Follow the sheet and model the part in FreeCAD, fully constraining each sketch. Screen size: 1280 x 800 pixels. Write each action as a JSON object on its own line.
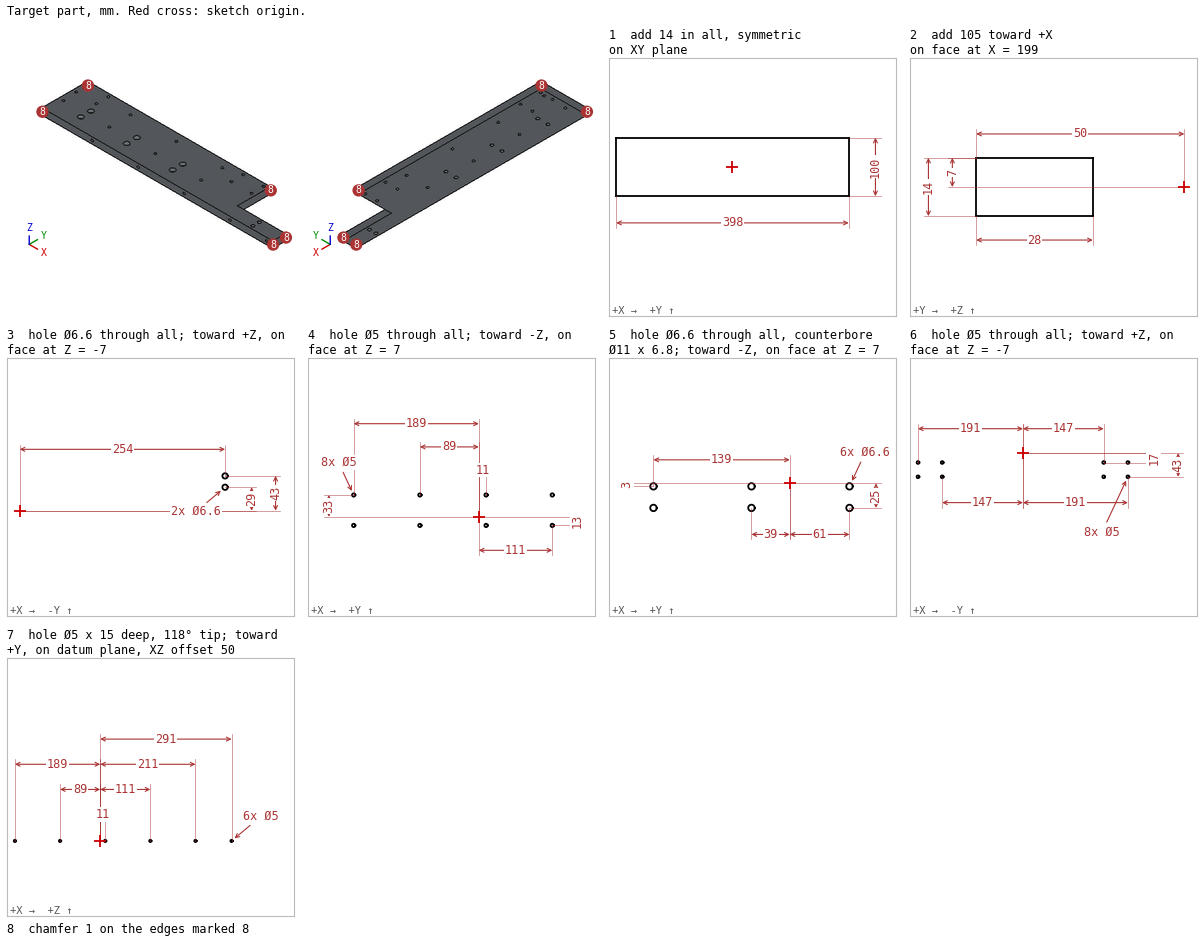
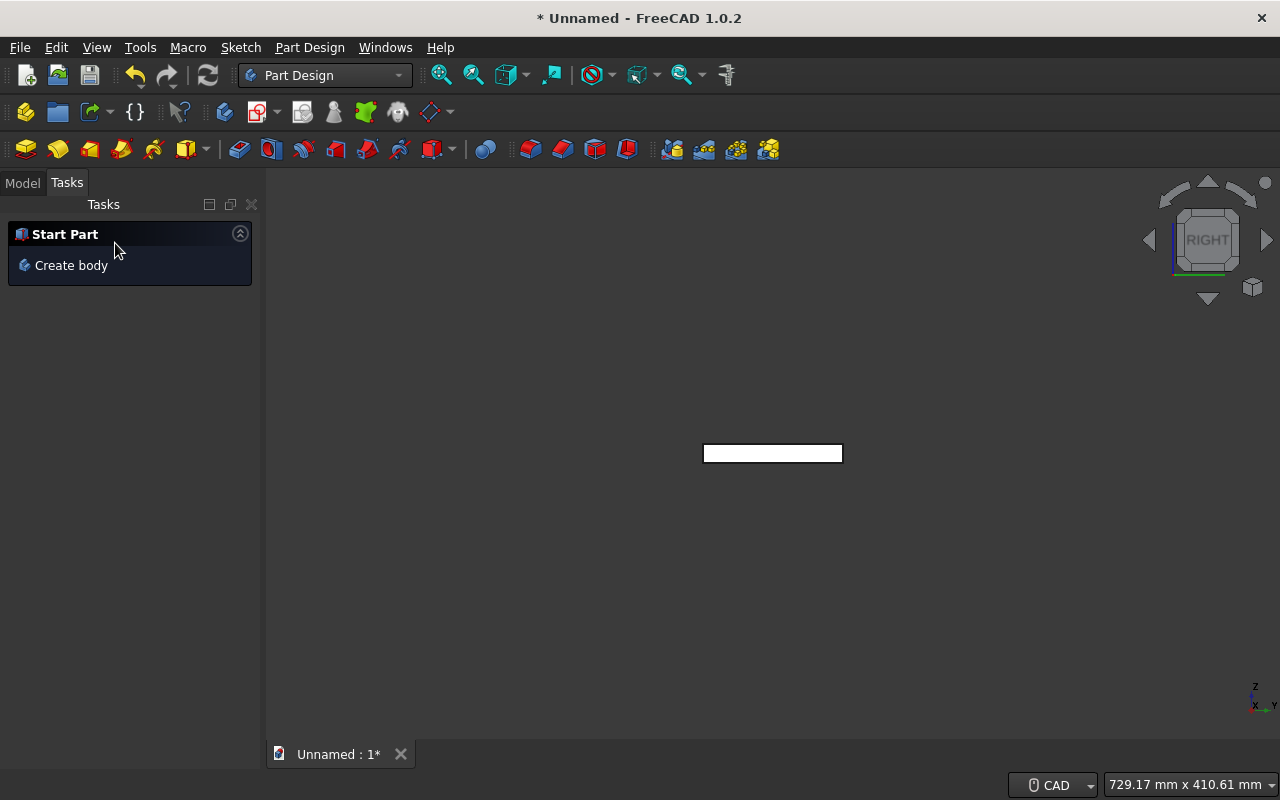
{"action": "key", "text": "v f"}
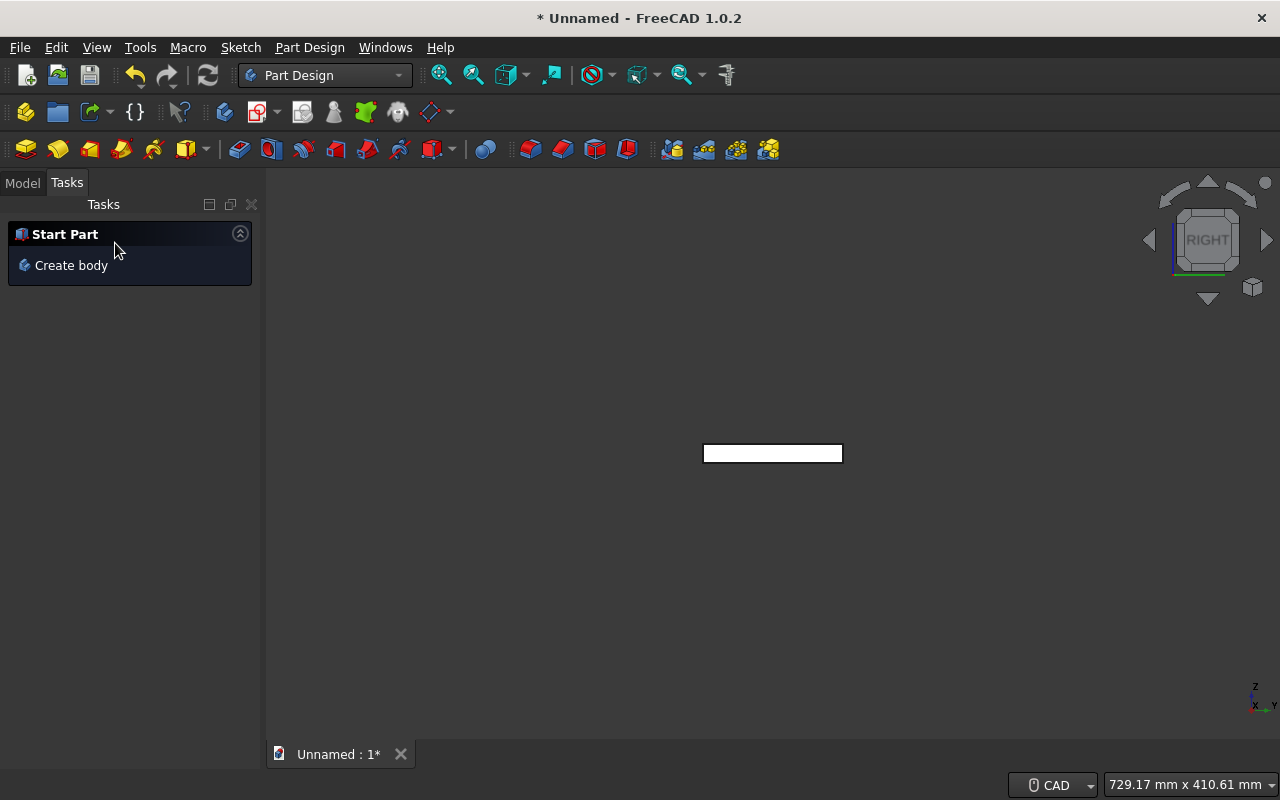
{"action": "left_click", "coordinate": [833, 452]}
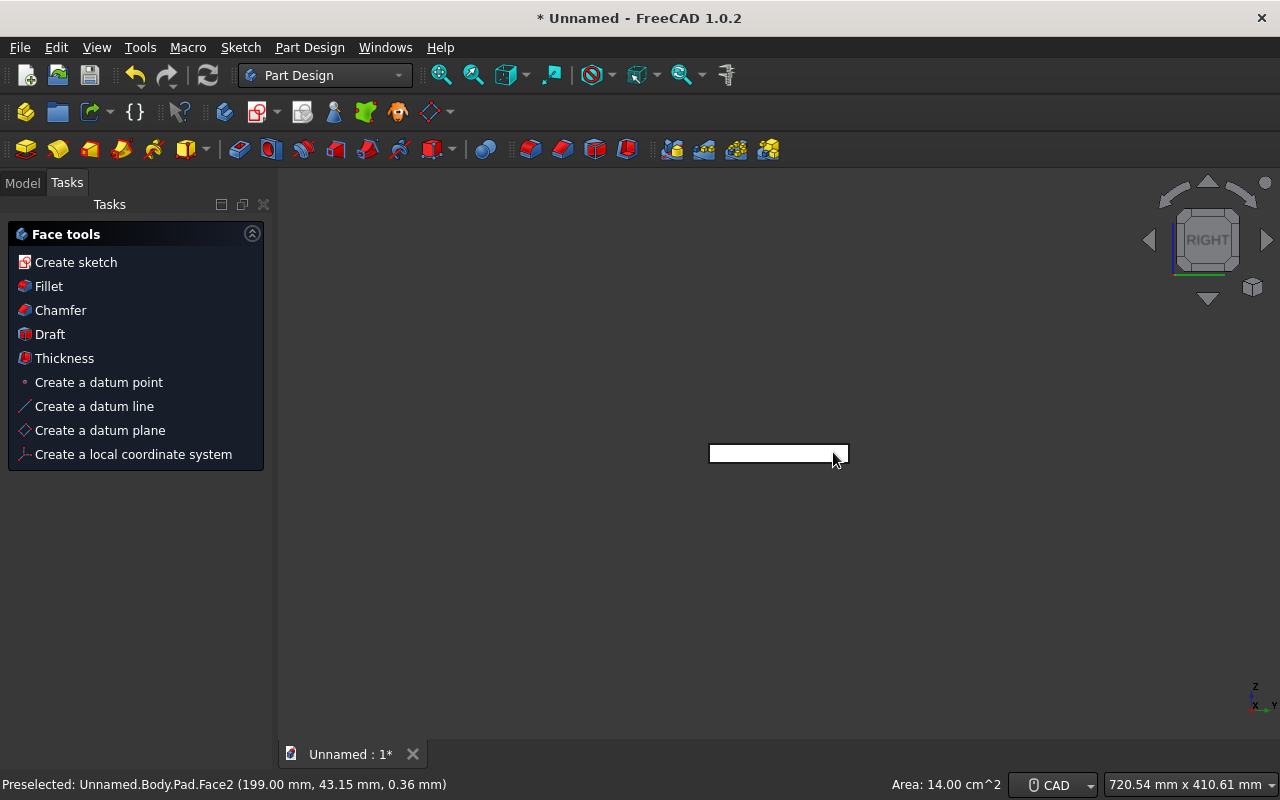
{"action": "left_click", "coordinate": [258, 112]}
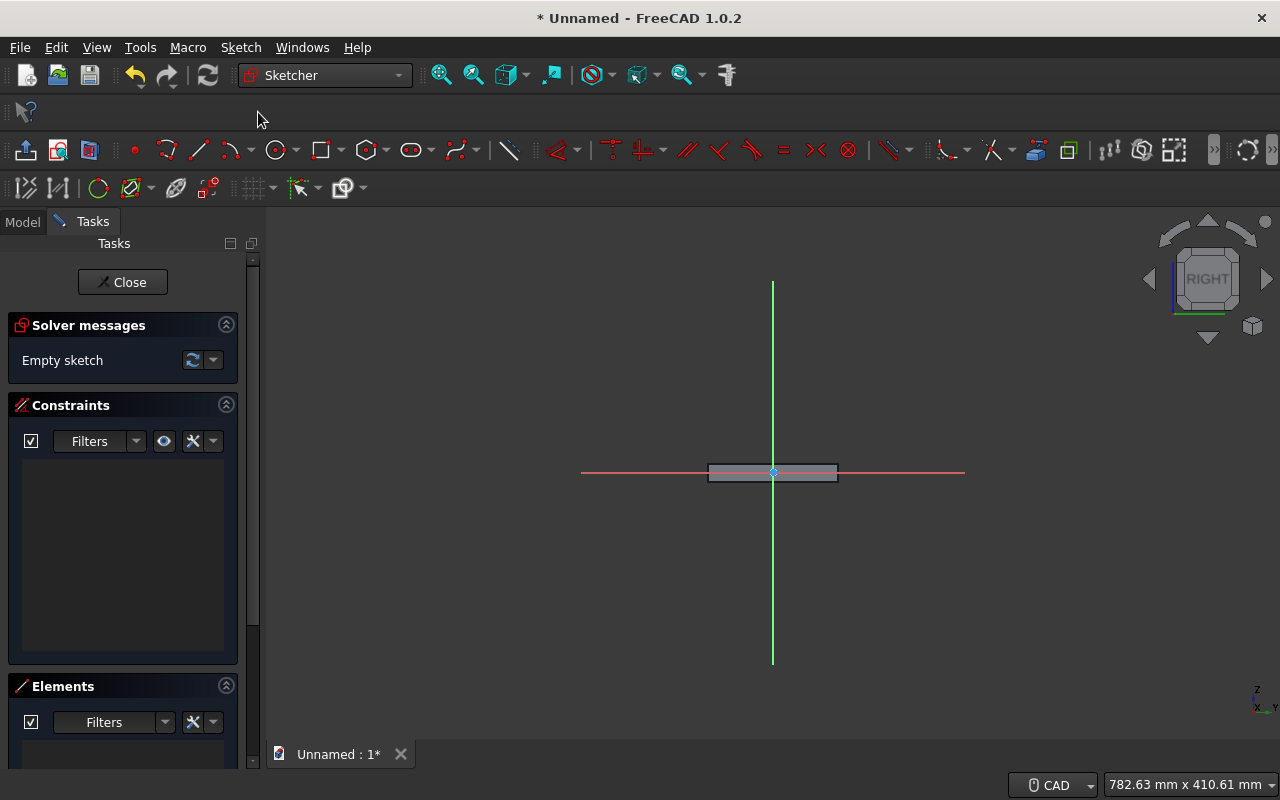
{"action": "scroll", "coordinate": [745, 473], "scroll_direction": "up", "scroll_amount": 11}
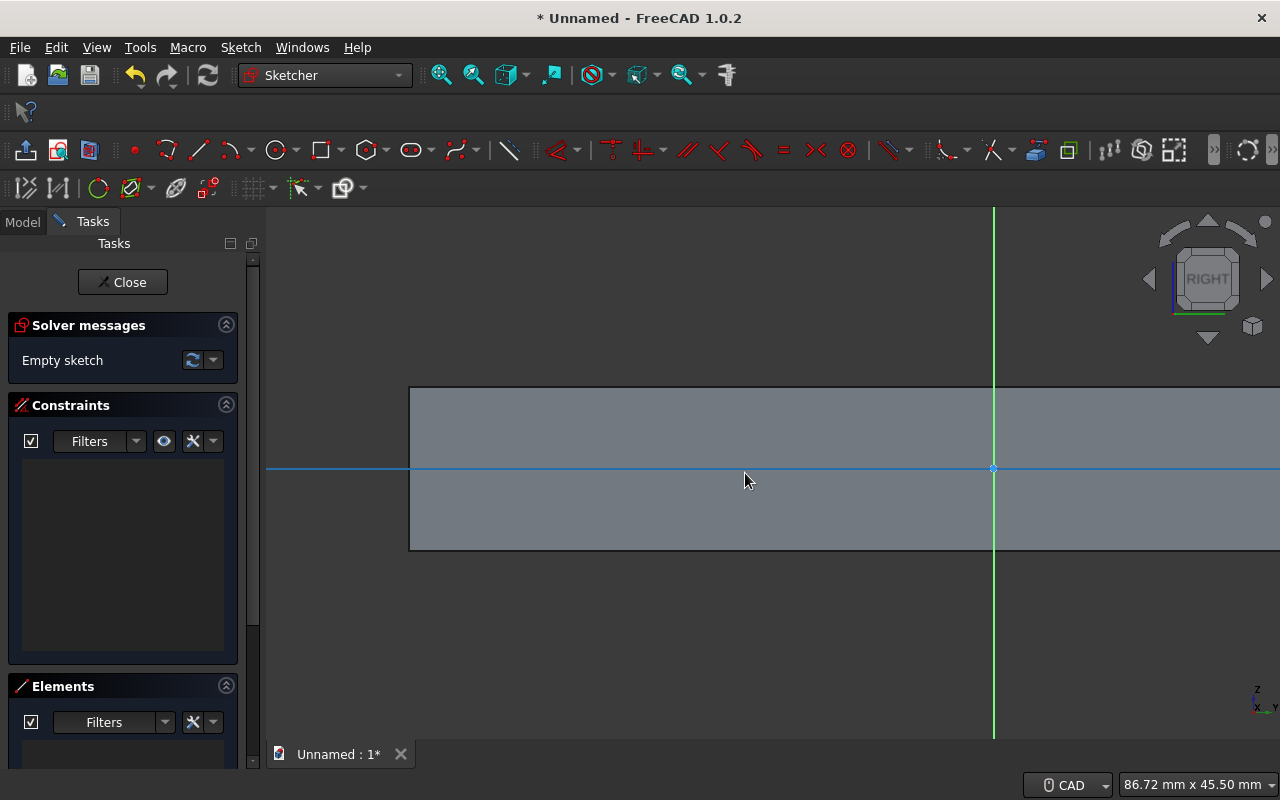
{"action": "key", "text": "g r"}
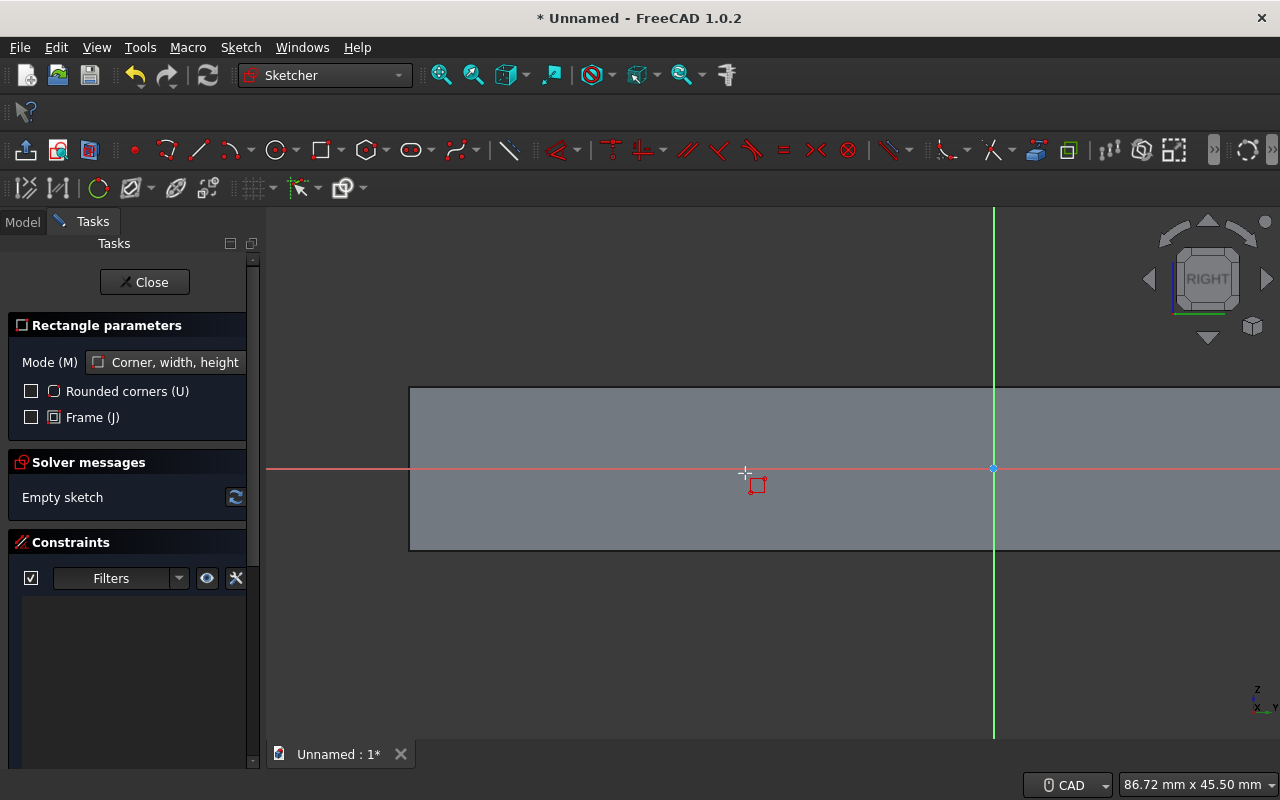
{"action": "left_click", "coordinate": [409, 387]}
{"action": "left_click", "coordinate": [737, 551]}
{"action": "key", "text": "Escape"}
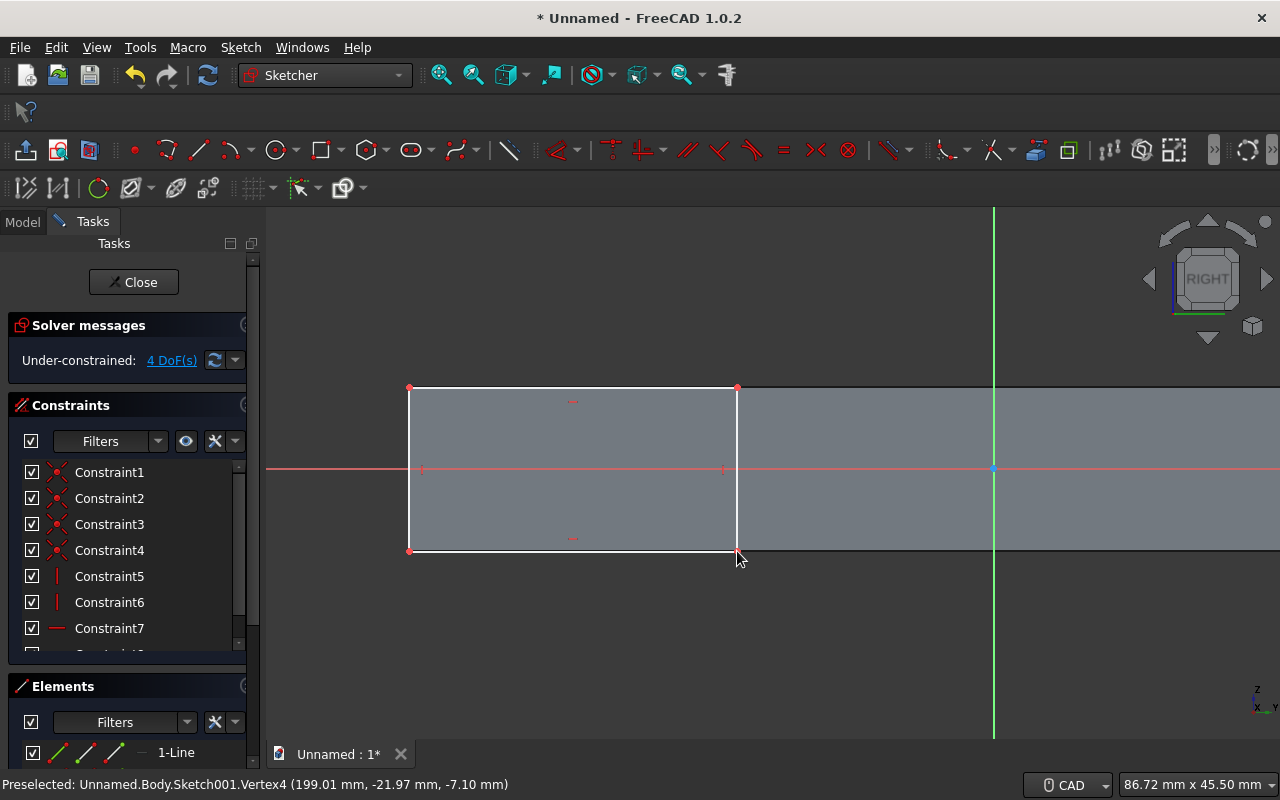
{"action": "key", "text": "d"}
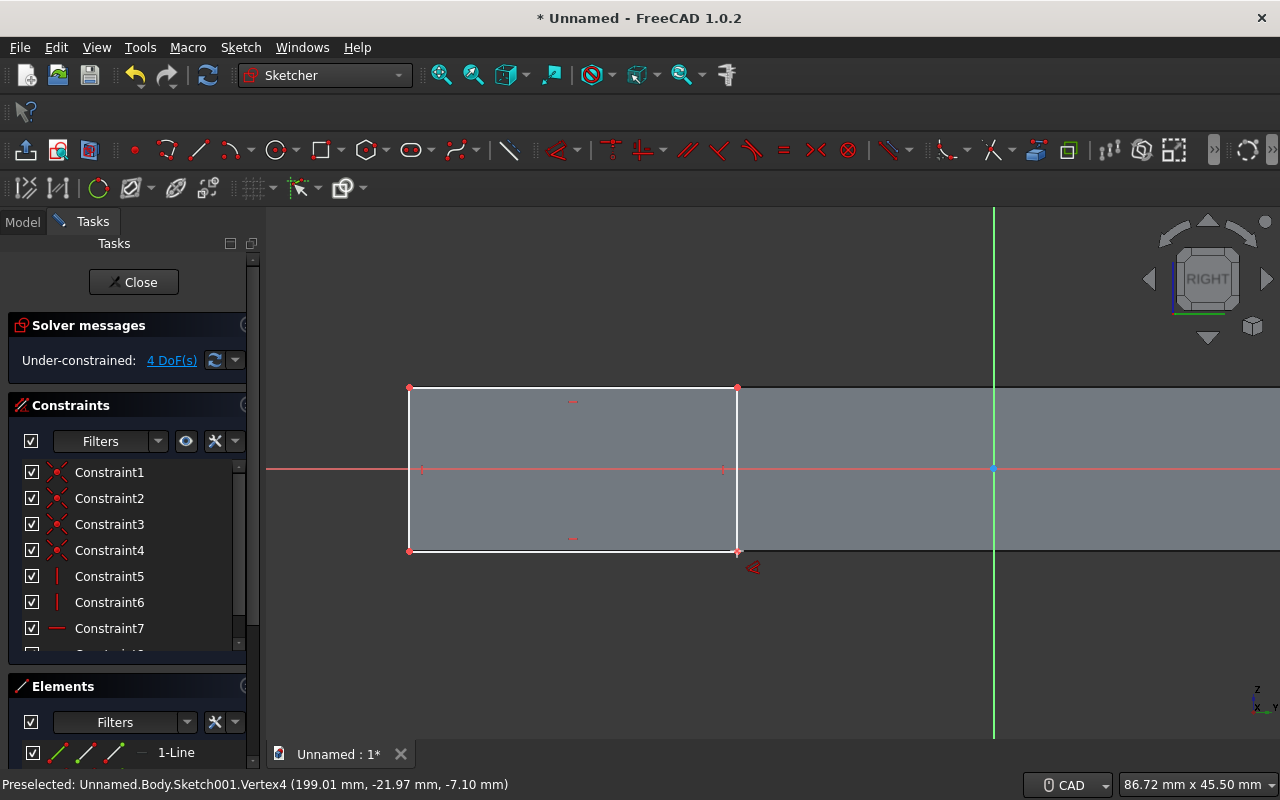
{"action": "left_click", "coordinate": [409, 437]}
{"action": "left_click", "coordinate": [375, 432]}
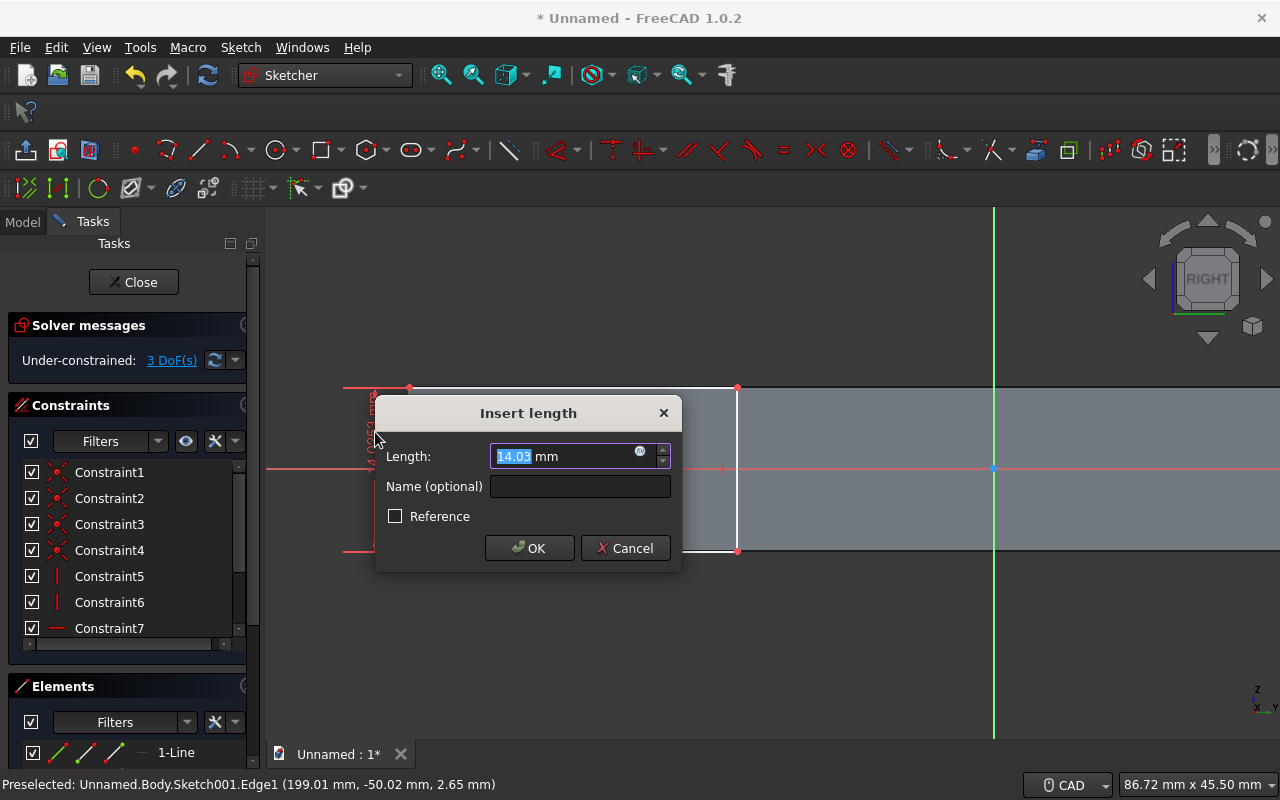
{"action": "type", "text": "14"}
{"action": "key", "text": "Return"}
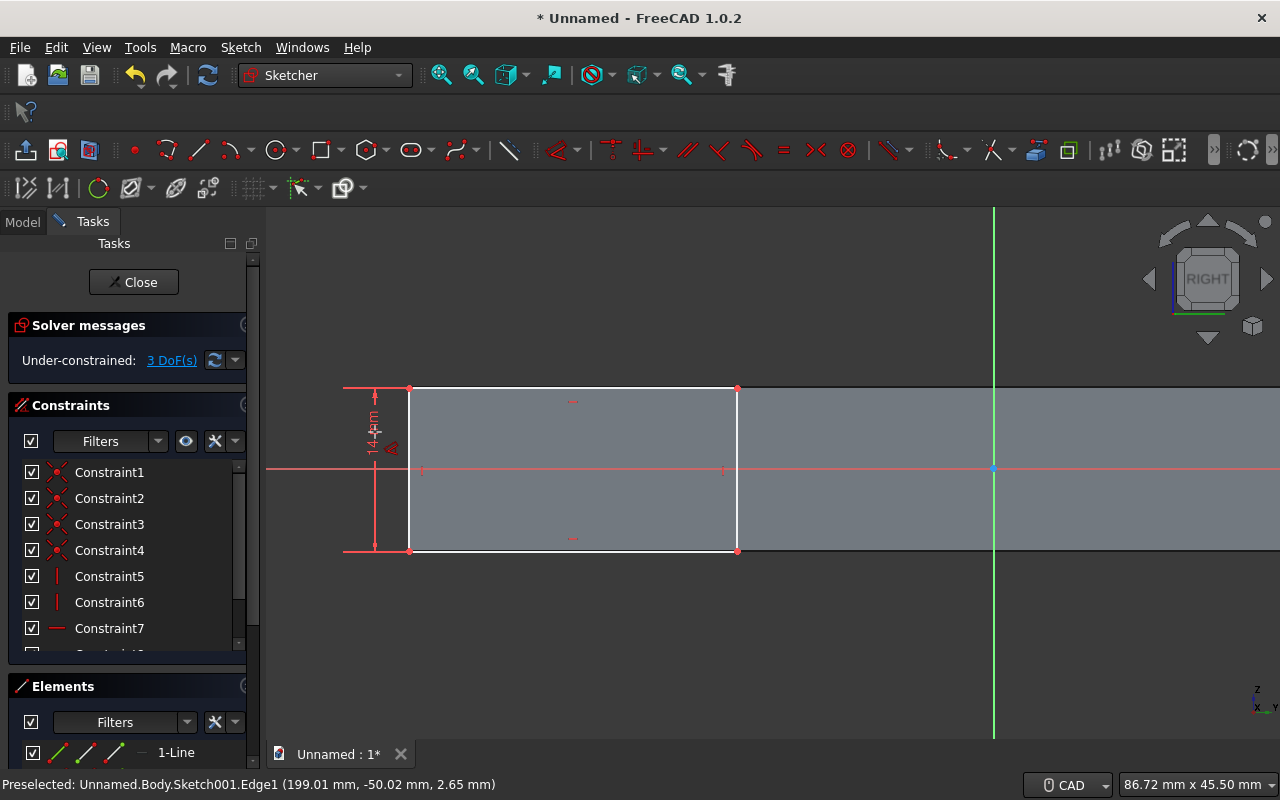
{"action": "left_click", "coordinate": [507, 552]}
{"action": "left_click", "coordinate": [573, 586]}